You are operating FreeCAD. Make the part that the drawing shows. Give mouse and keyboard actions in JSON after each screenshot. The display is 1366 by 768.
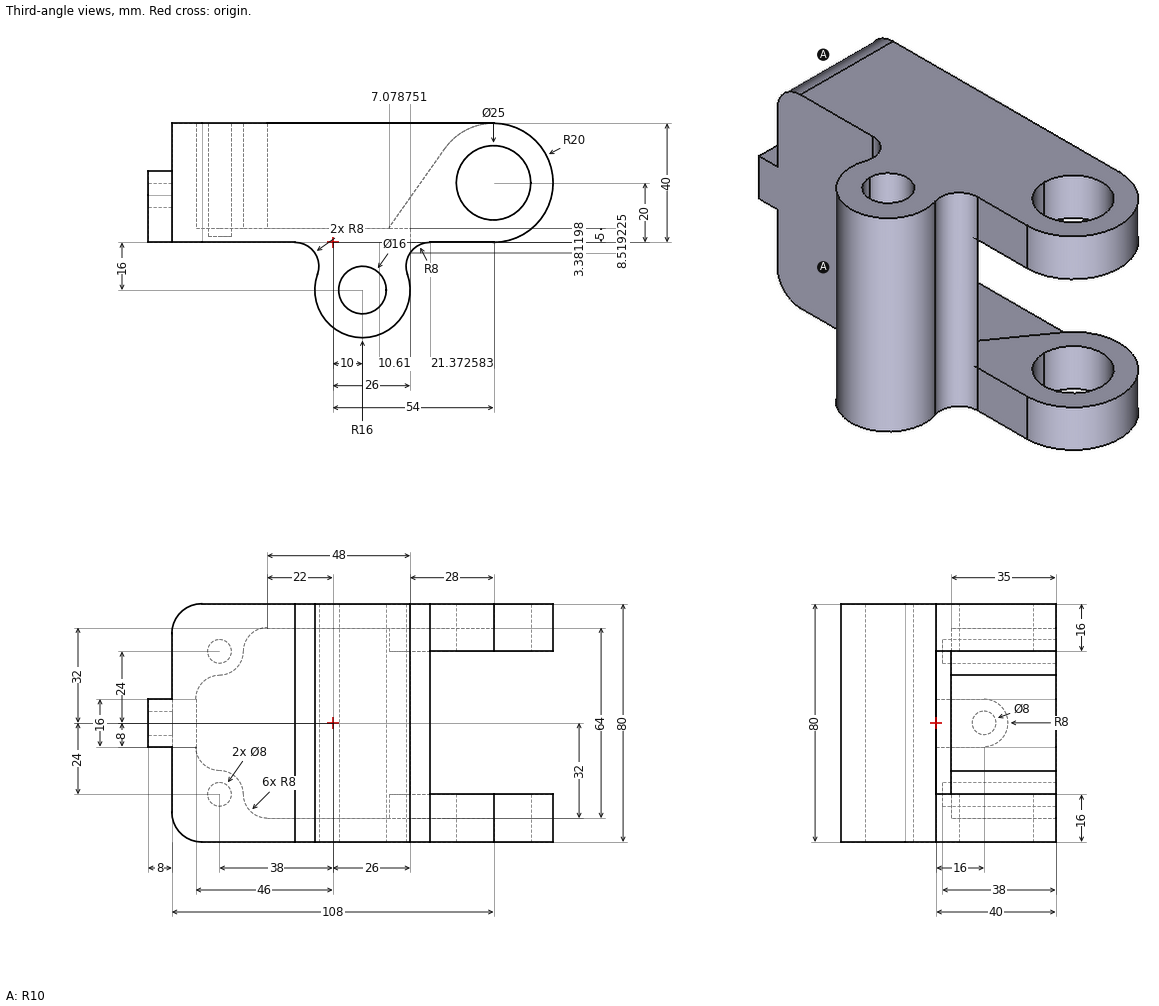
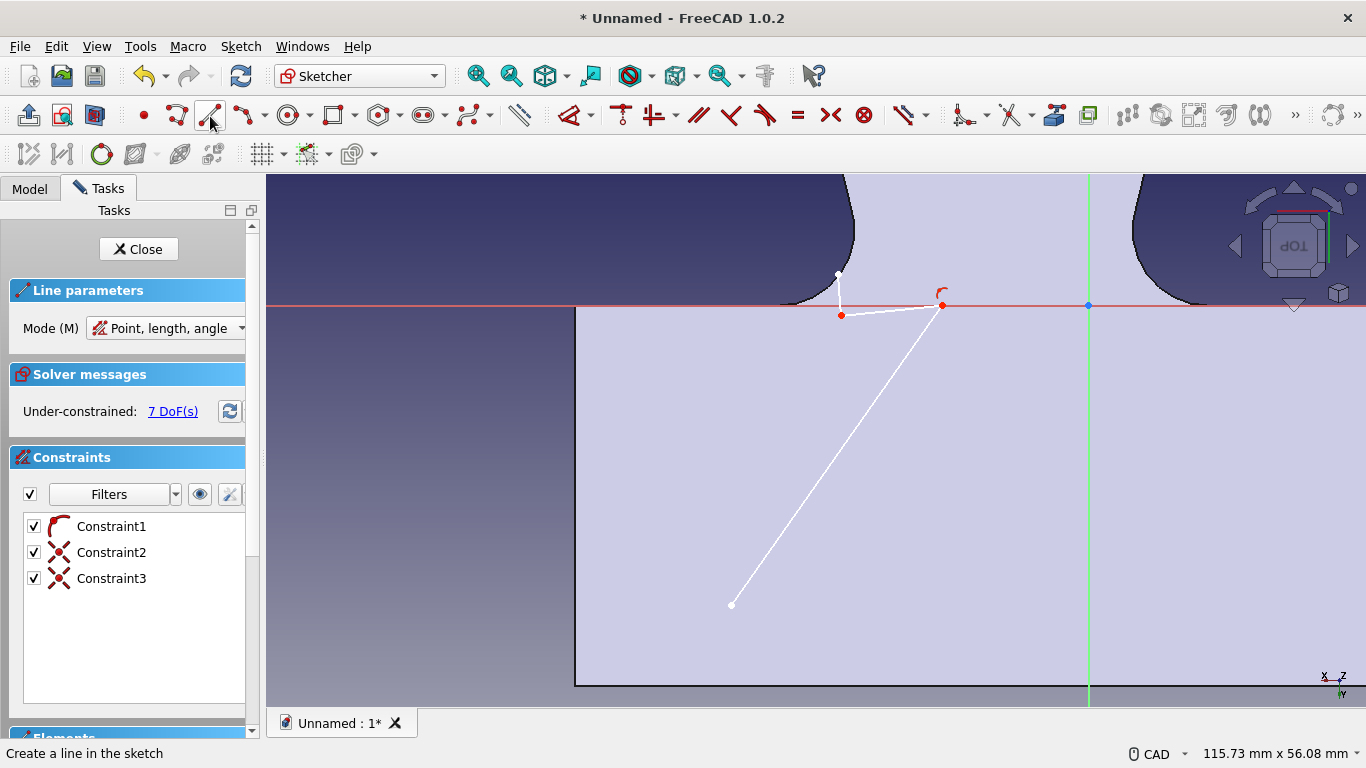
{"action": "left_click", "coordinate": [778, 306]}
{"action": "left_click", "coordinate": [575, 315]}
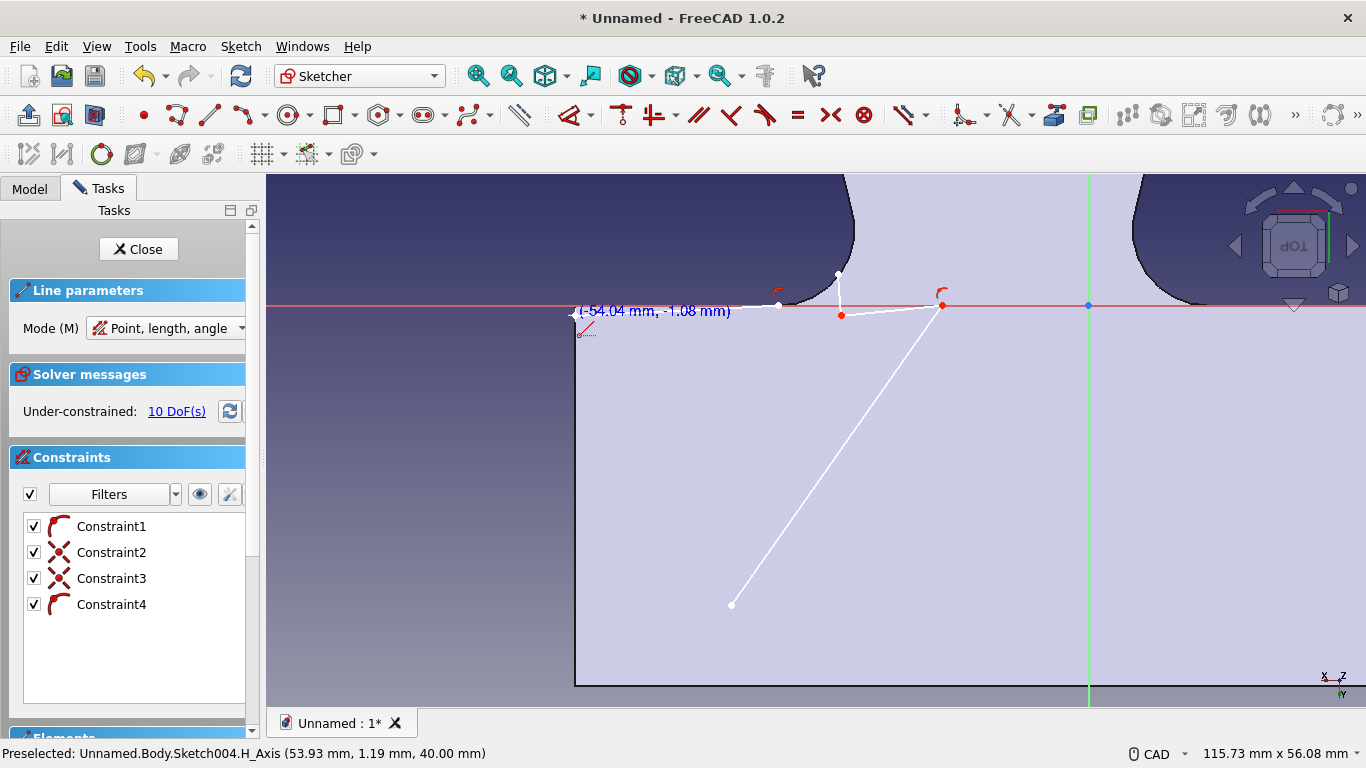
{"action": "key", "text": "g 3 a"}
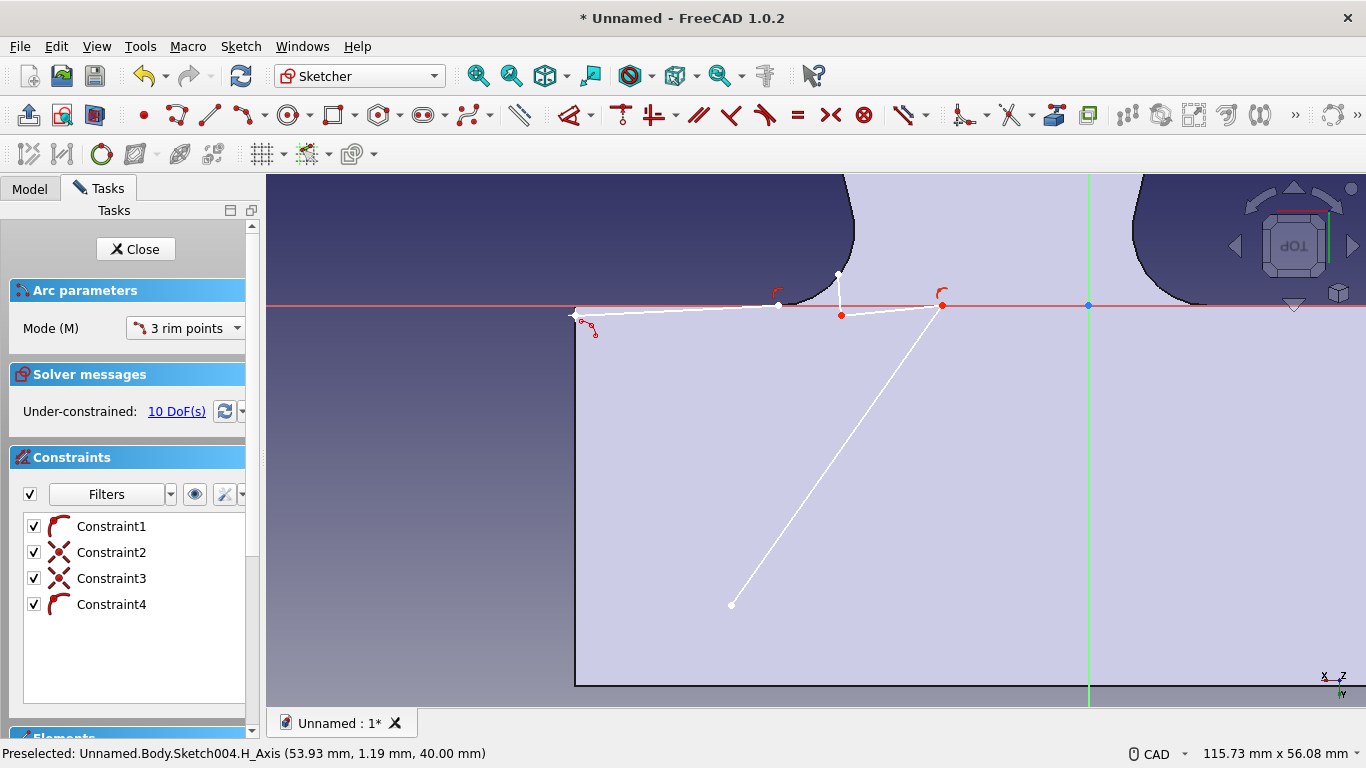
{"action": "left_click", "coordinate": [838, 275]}
{"action": "left_click", "coordinate": [778, 306]}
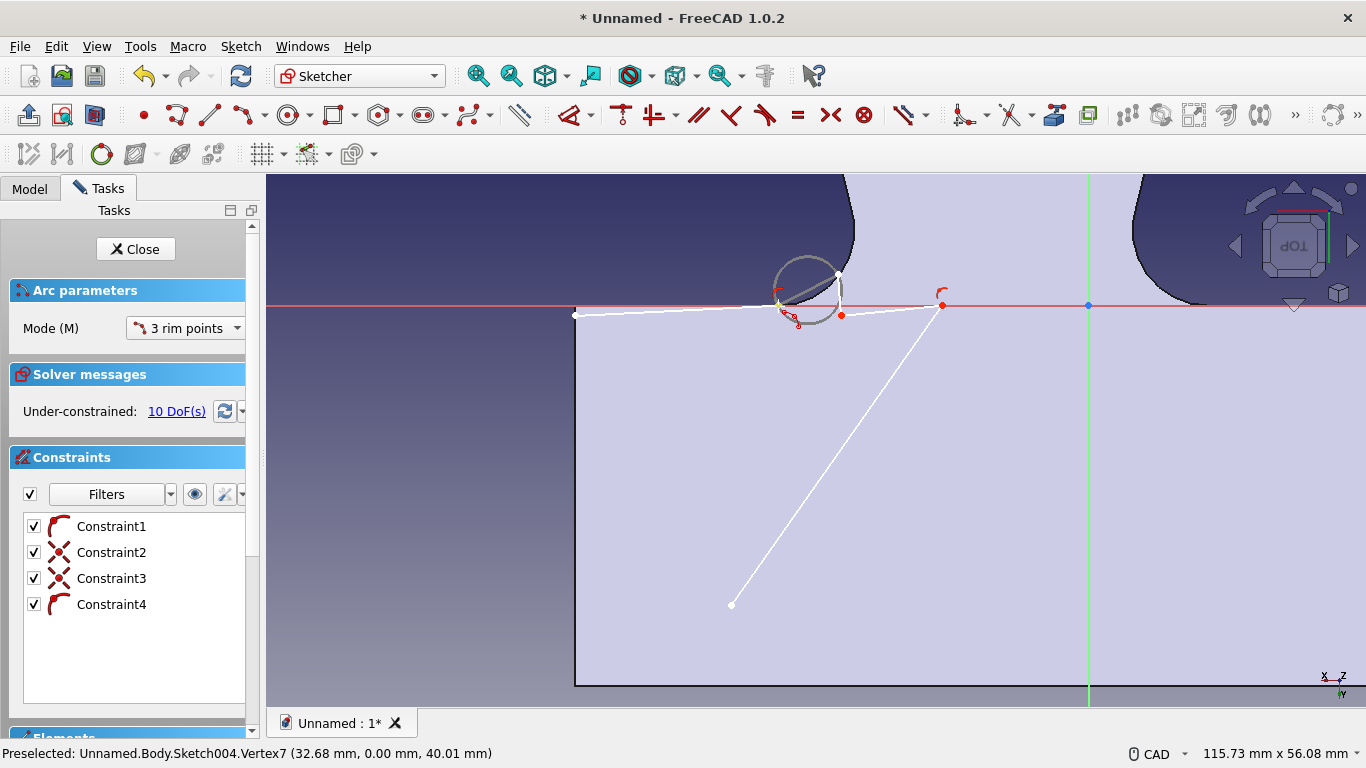
{"action": "scroll", "coordinate": [813, 297], "scroll_direction": "up", "scroll_amount": 4}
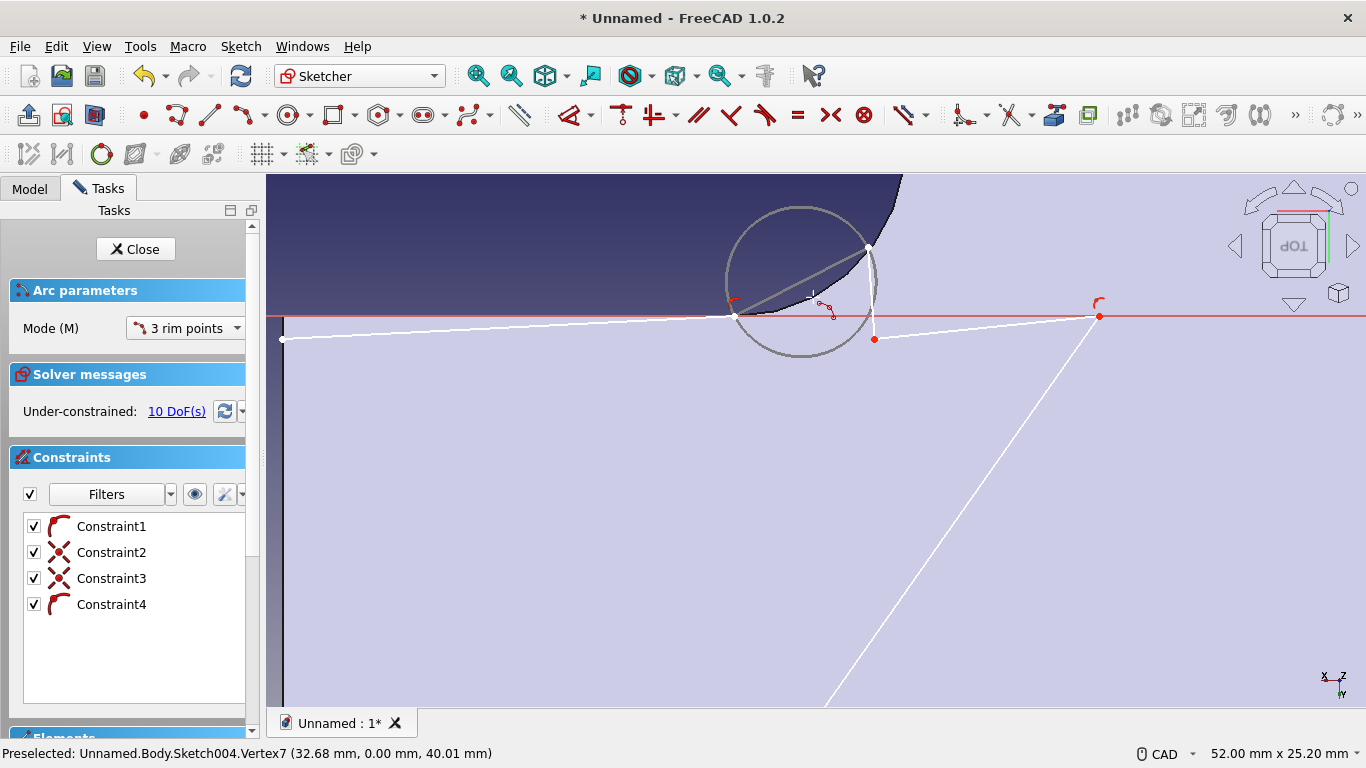
{"action": "left_click", "coordinate": [813, 297]}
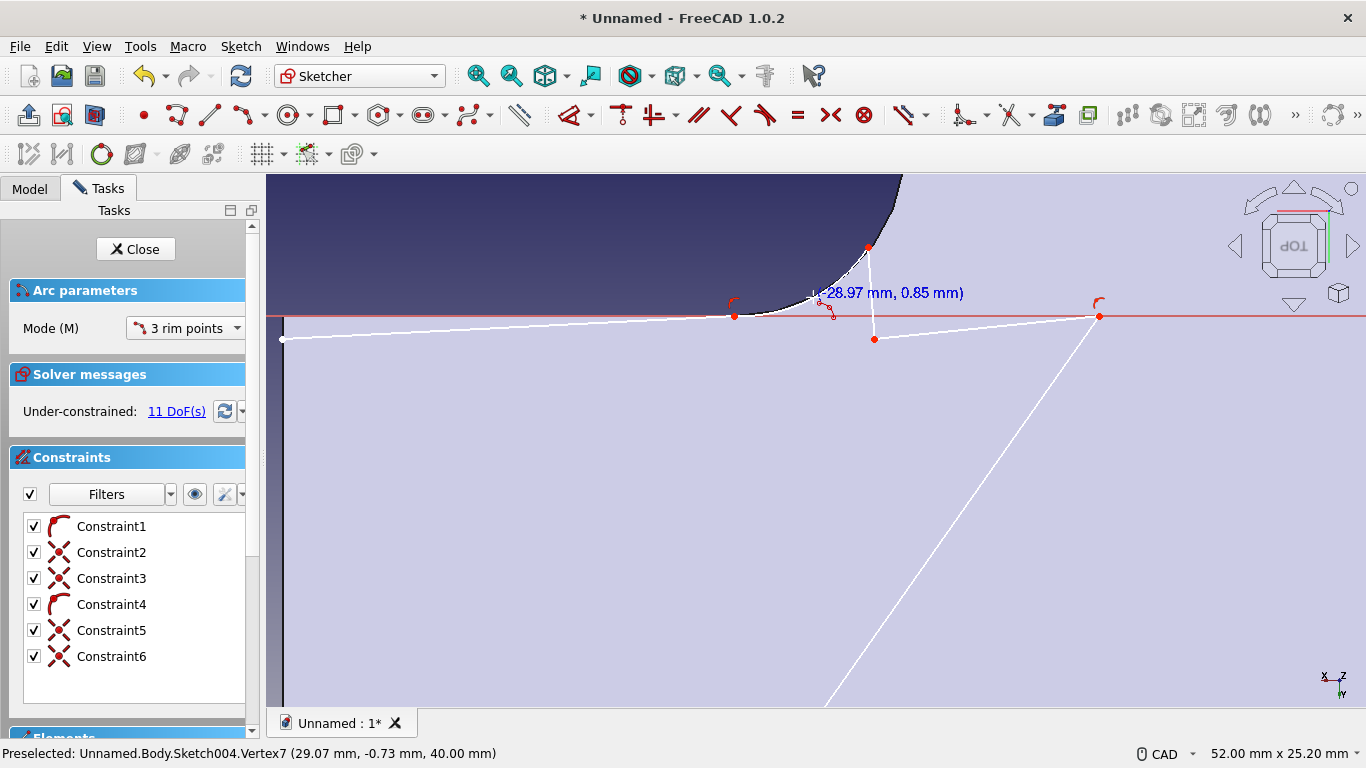
{"action": "scroll", "coordinate": [813, 299], "scroll_direction": "down", "scroll_amount": 4}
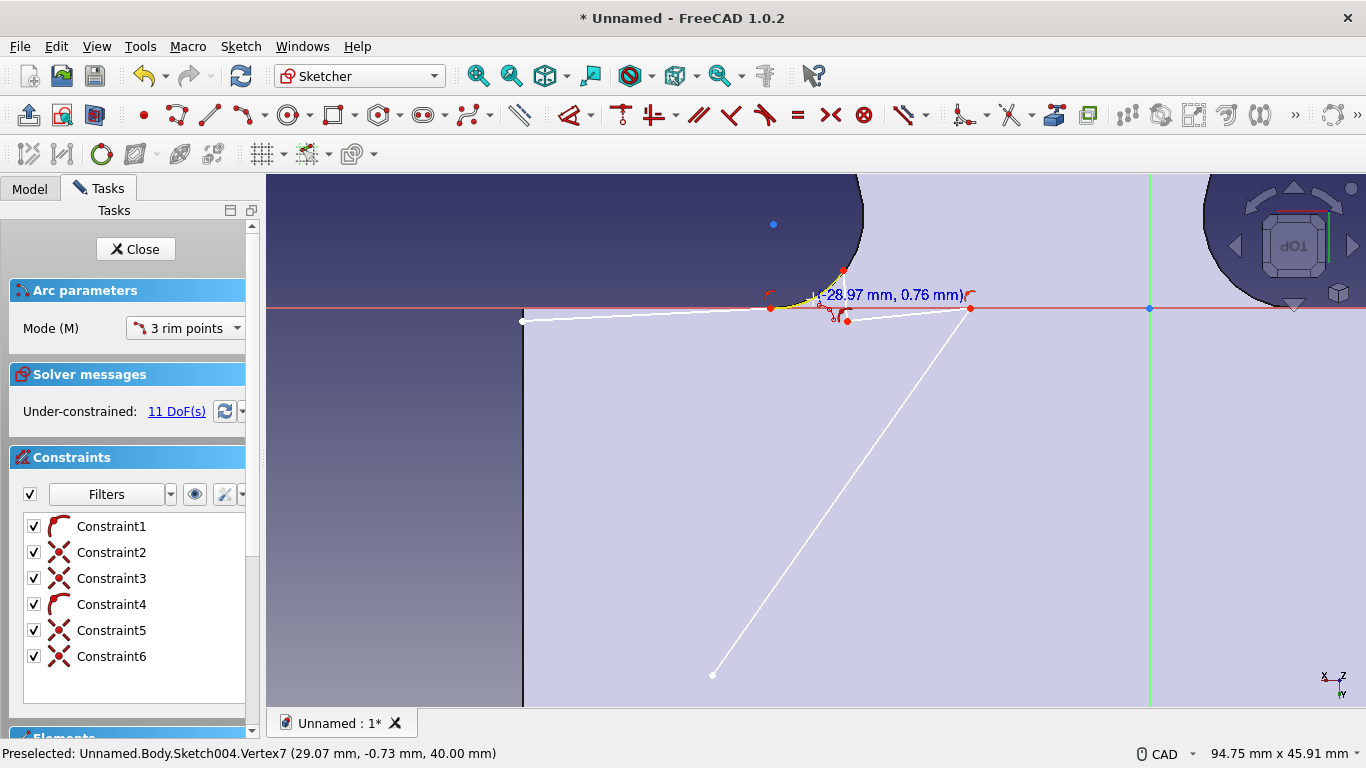
{"action": "left_click", "coordinate": [575, 317]}
{"action": "left_click", "coordinate": [731, 607]}
{"action": "left_click", "coordinate": [407, 584]}
{"action": "key", "text": "Escape"}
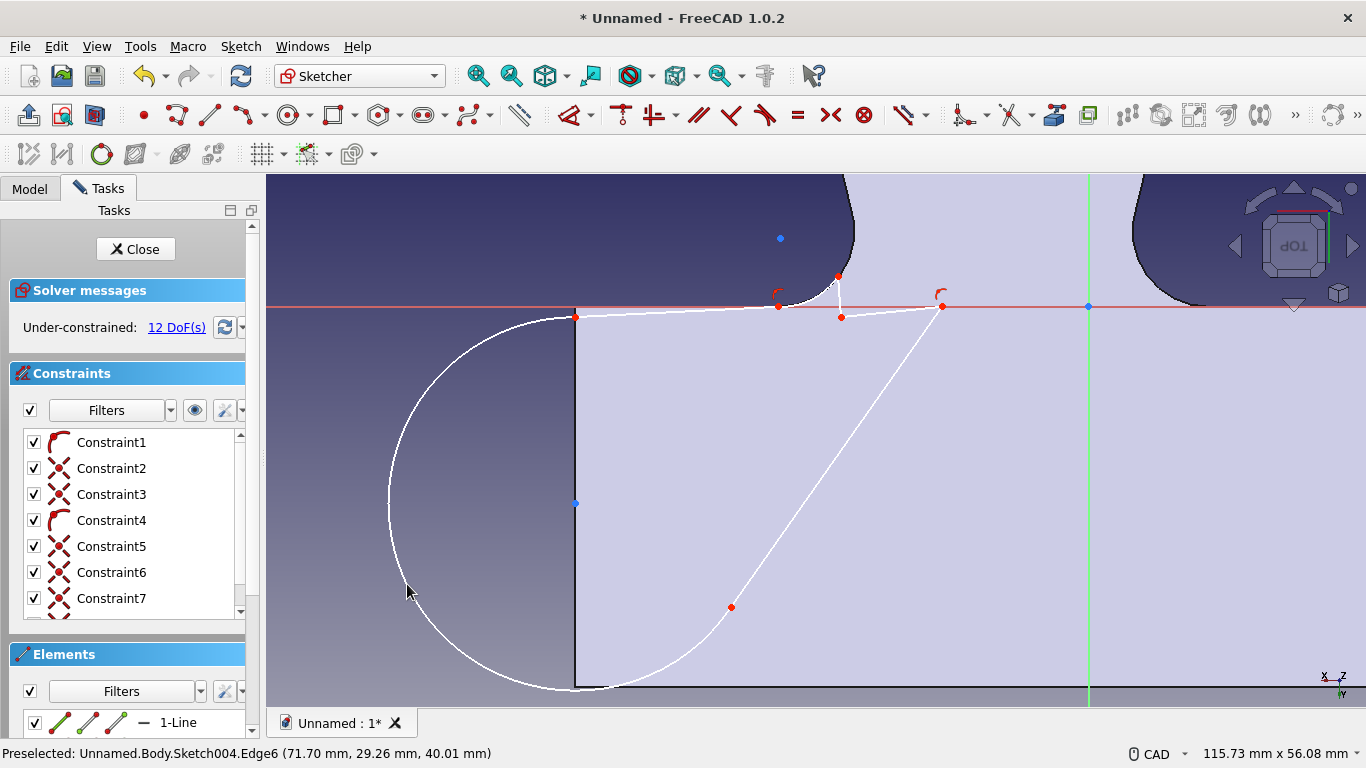
{"action": "left_click", "coordinate": [794, 517]}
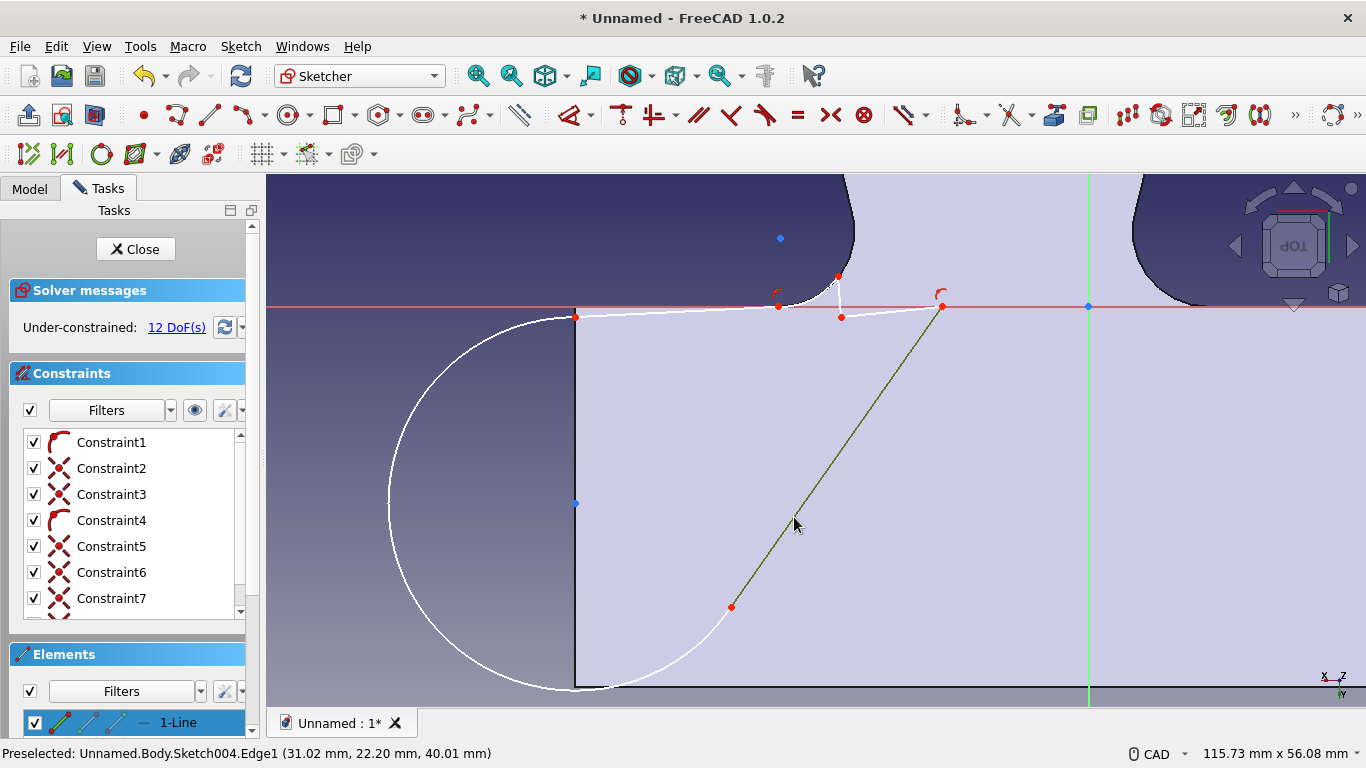
{"action": "left_click", "coordinate": [399, 443]}